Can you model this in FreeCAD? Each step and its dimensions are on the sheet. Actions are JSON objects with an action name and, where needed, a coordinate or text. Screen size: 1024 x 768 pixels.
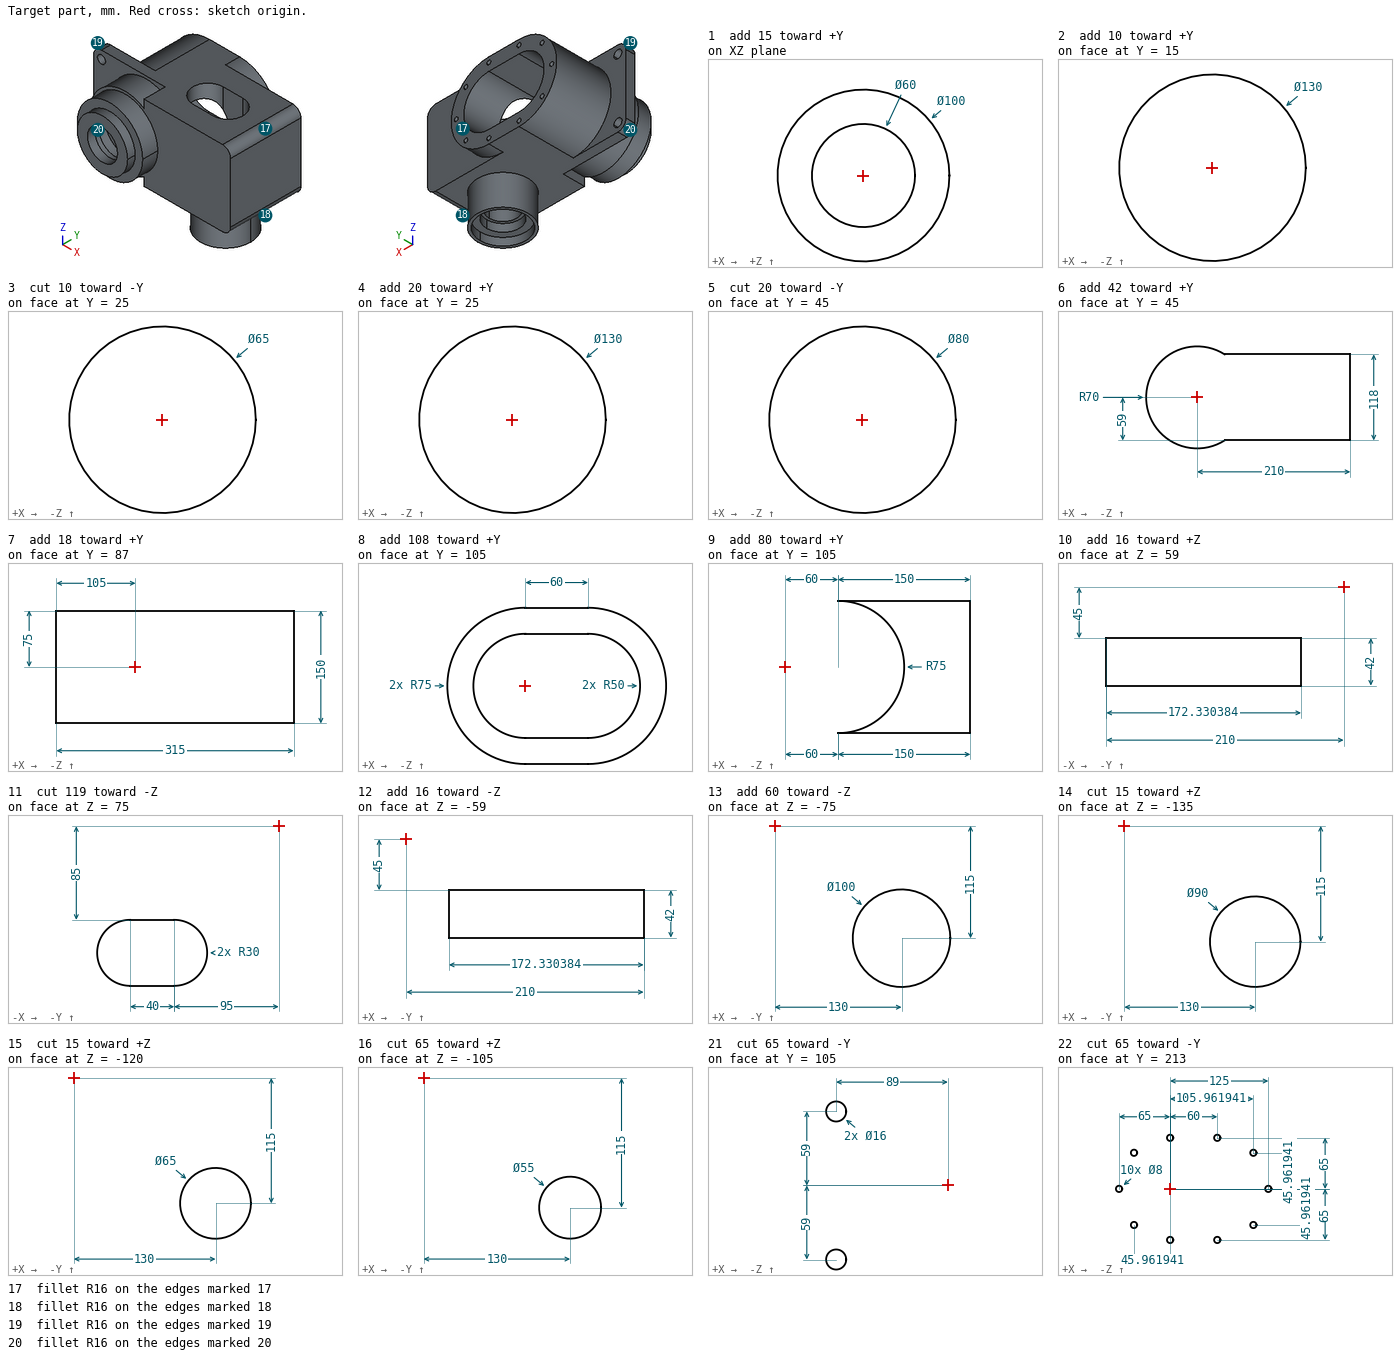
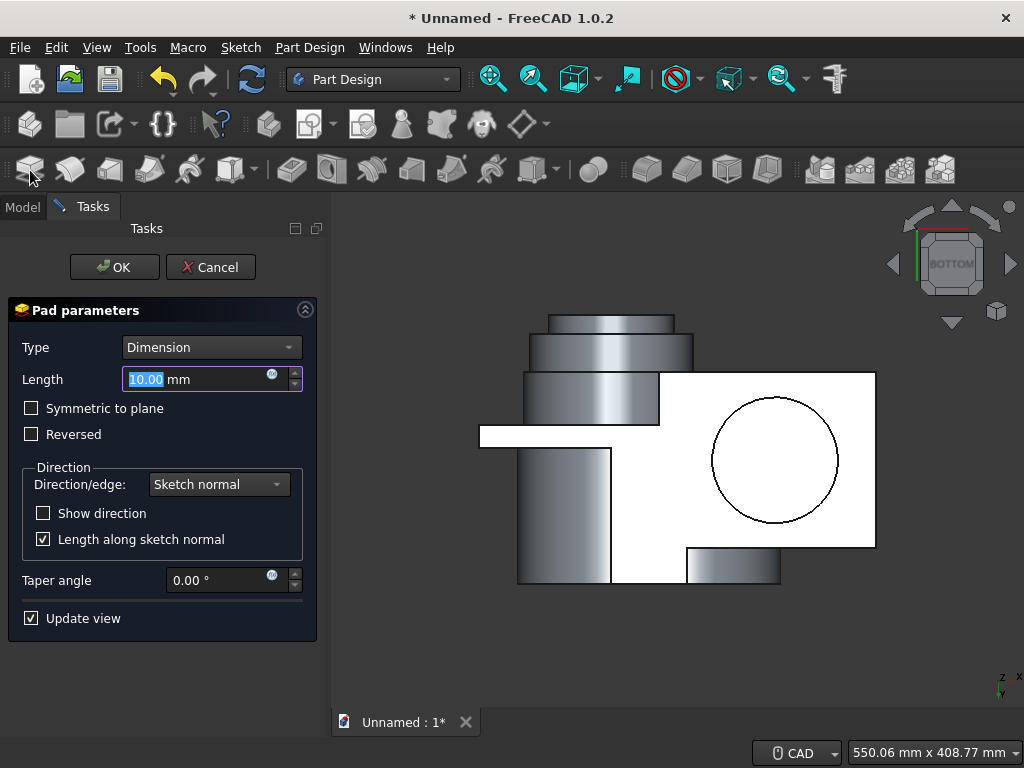
{"action": "type", "text": "60"}
{"action": "key", "text": "Tab"}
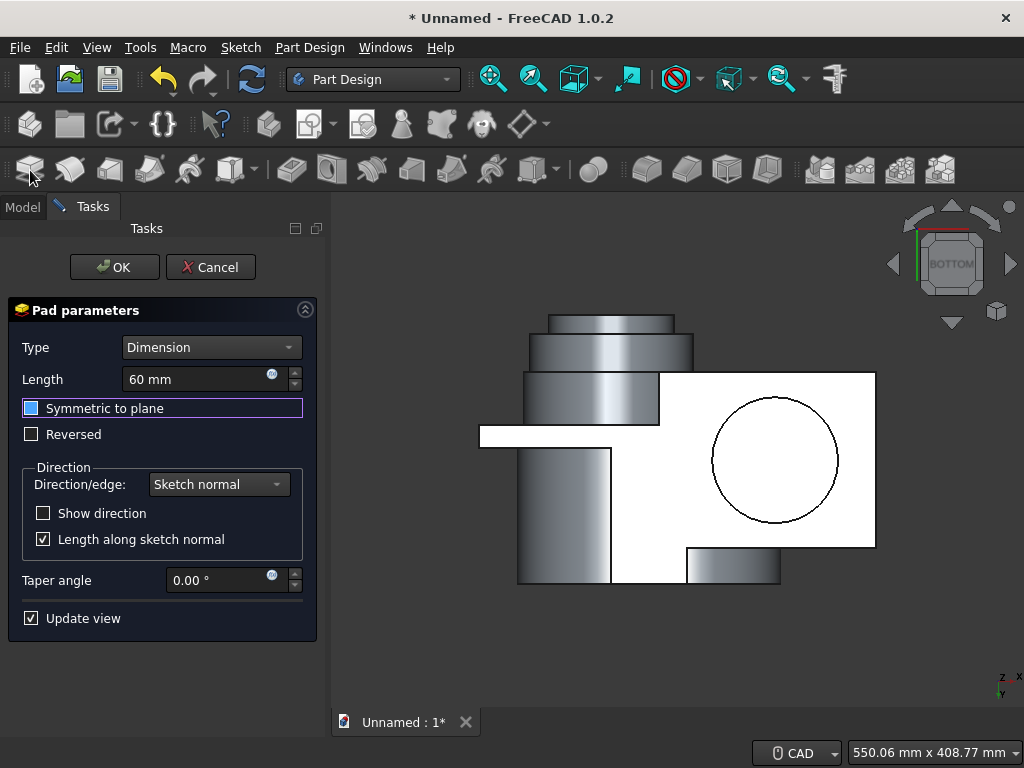
{"action": "left_click", "coordinate": [115, 267]}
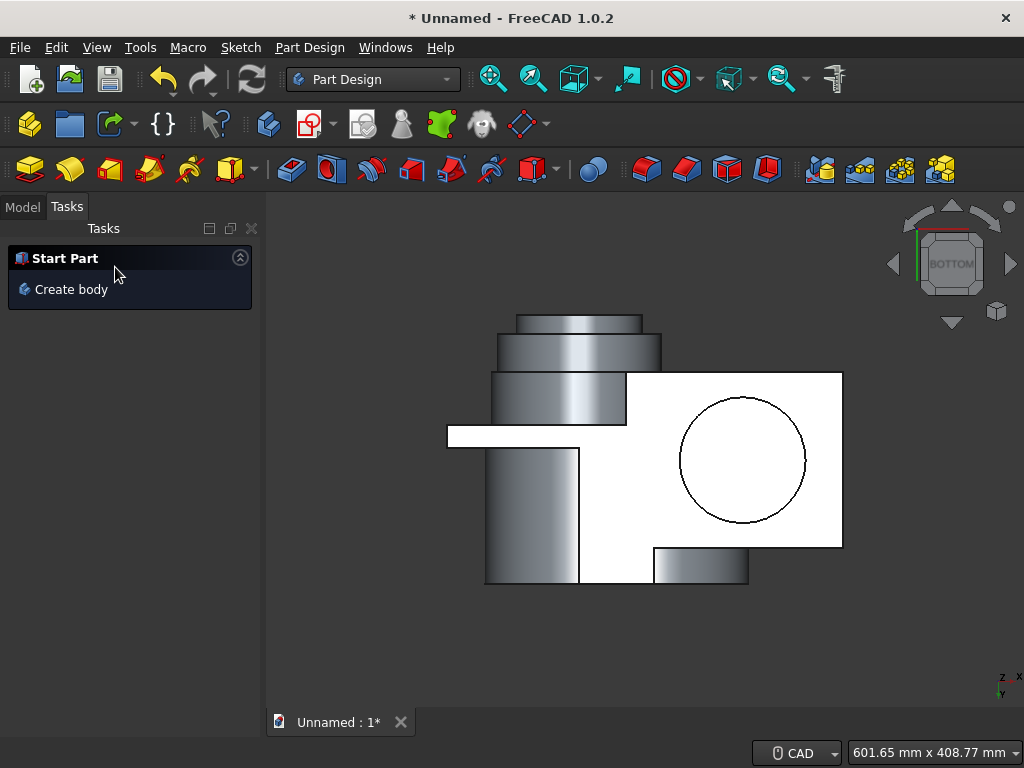
{"action": "left_click", "coordinate": [743, 459]}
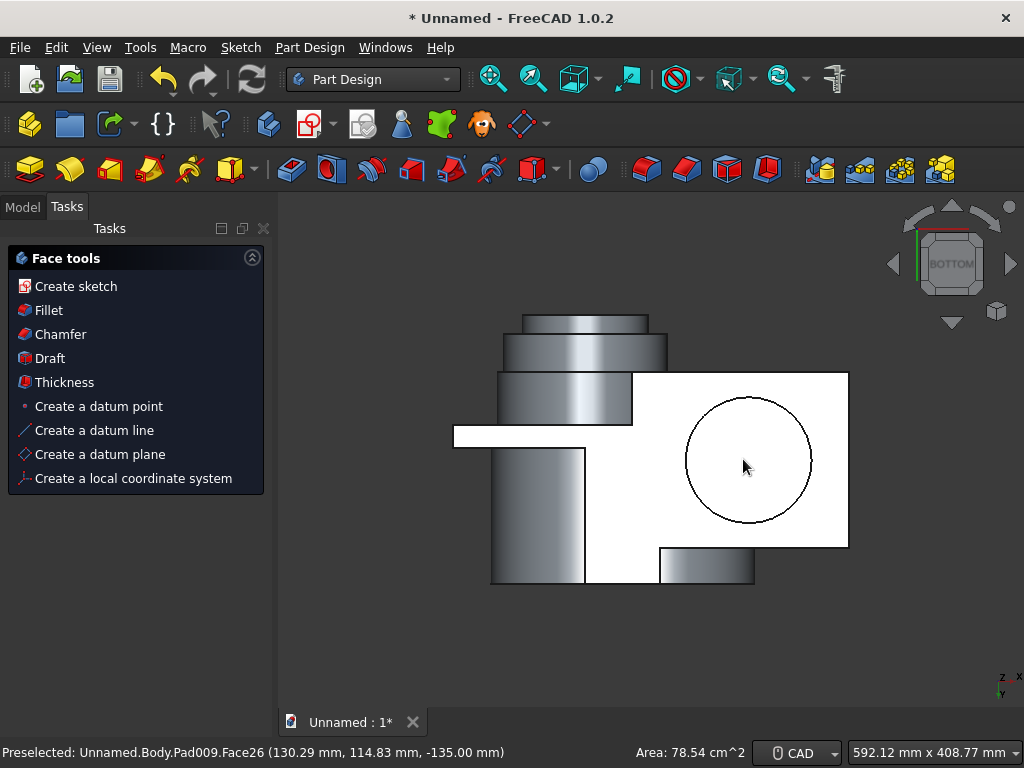
{"action": "left_click", "coordinate": [310, 124]}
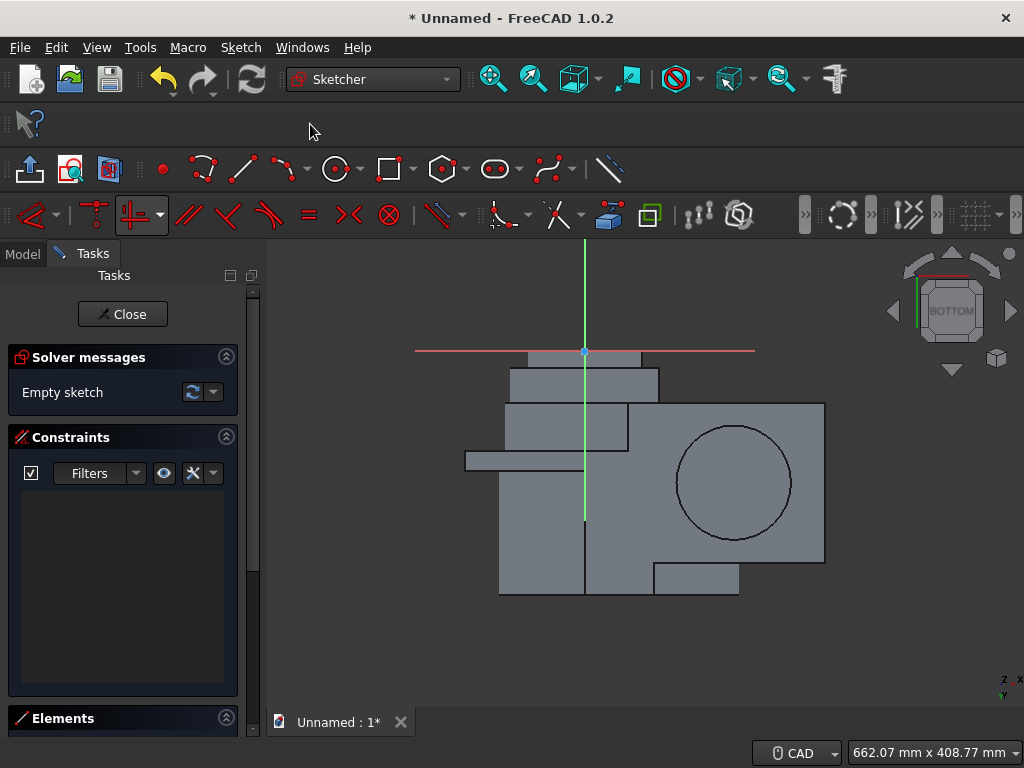
{"action": "scroll", "coordinate": [859, 381], "scroll_direction": "up", "scroll_amount": 2}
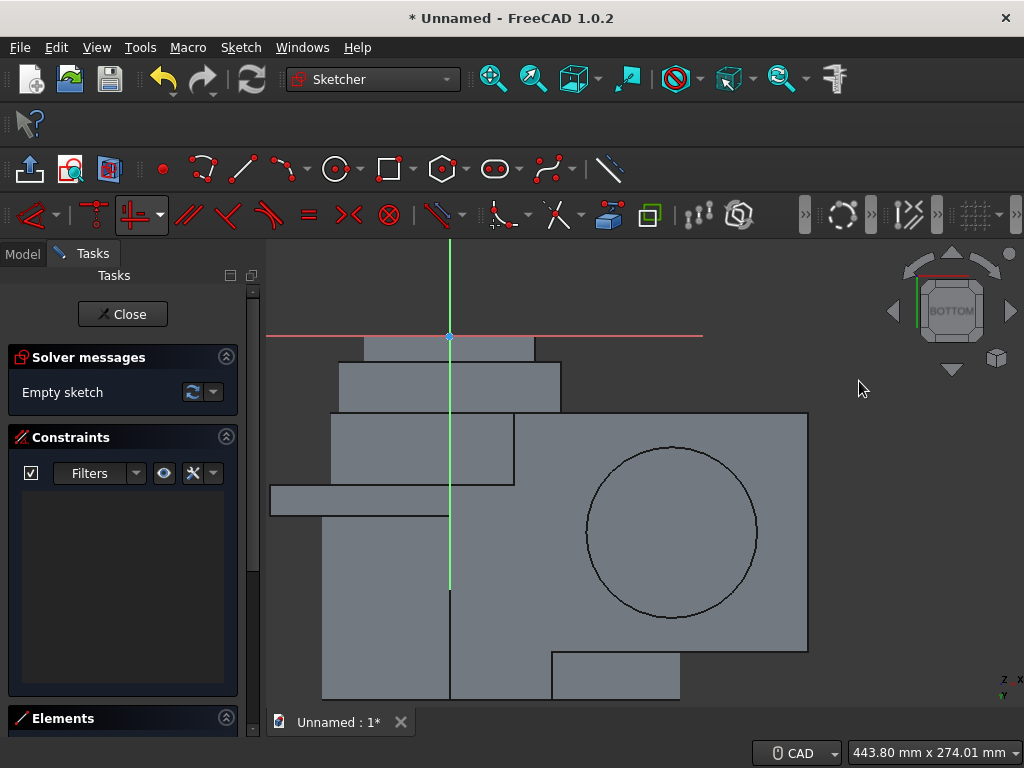
{"action": "left_click", "coordinate": [336, 170]}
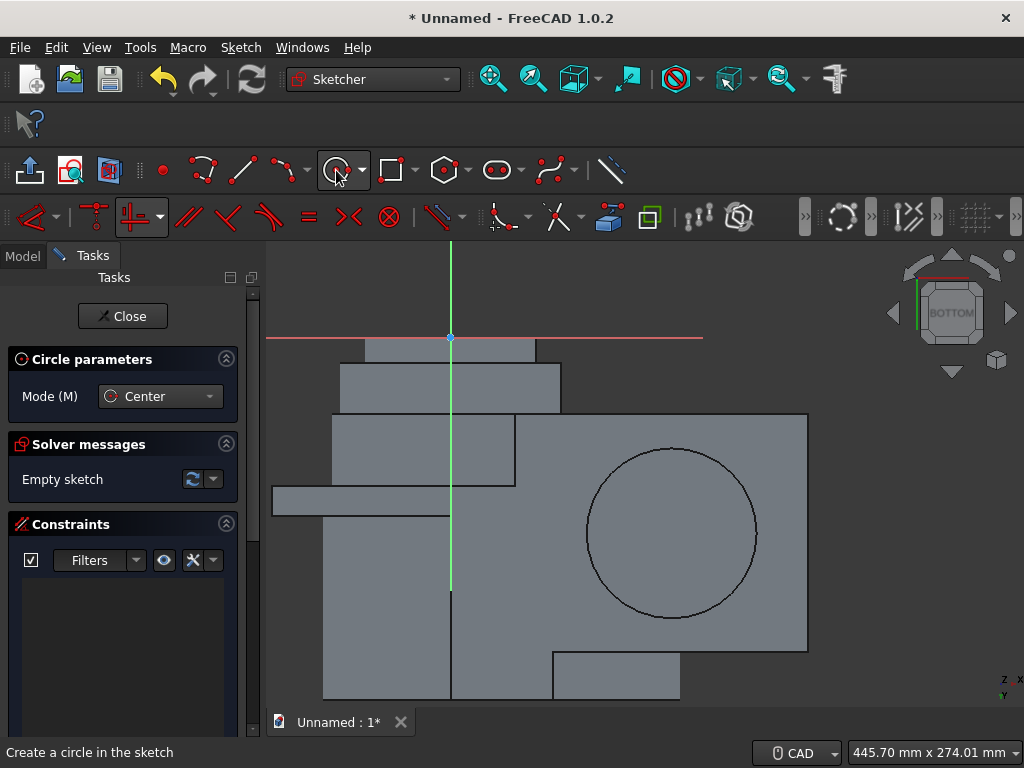
{"action": "left_click", "coordinate": [672, 533]}
{"action": "mouse_move", "coordinate": [726, 479]}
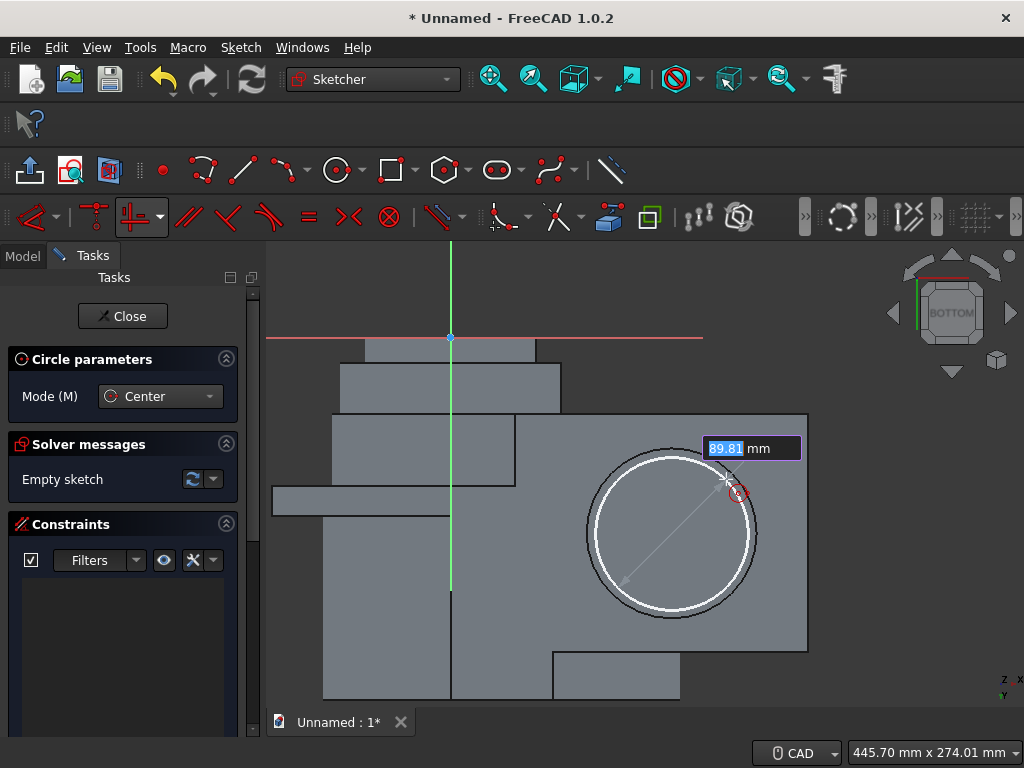
{"action": "type", "text": "90"}
{"action": "key", "text": "Return"}
{"action": "key", "text": "Escape"}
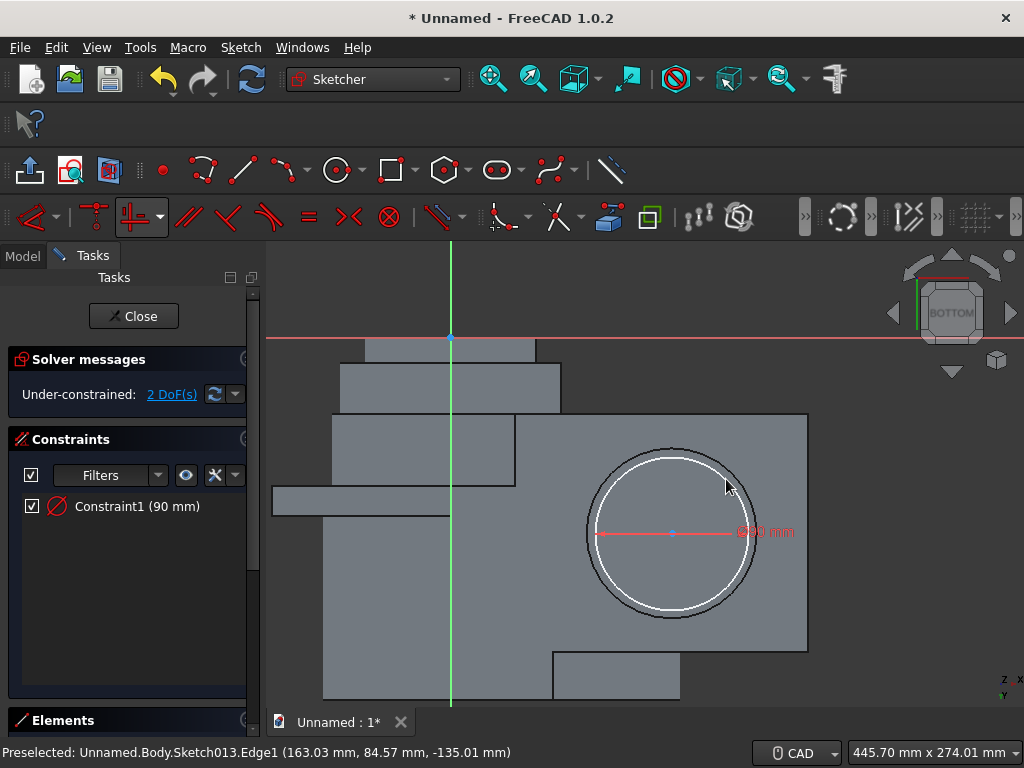
{"action": "left_click", "coordinate": [32, 218]}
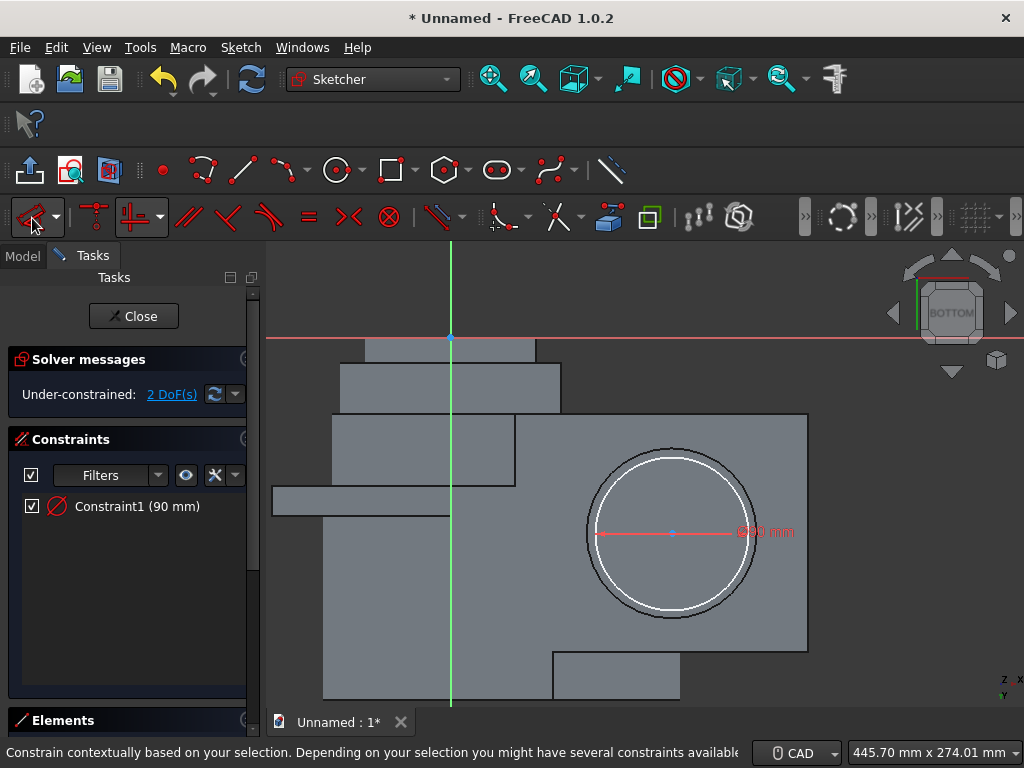
{"action": "left_click", "coordinate": [672, 534]}
{"action": "left_click", "coordinate": [561, 304]}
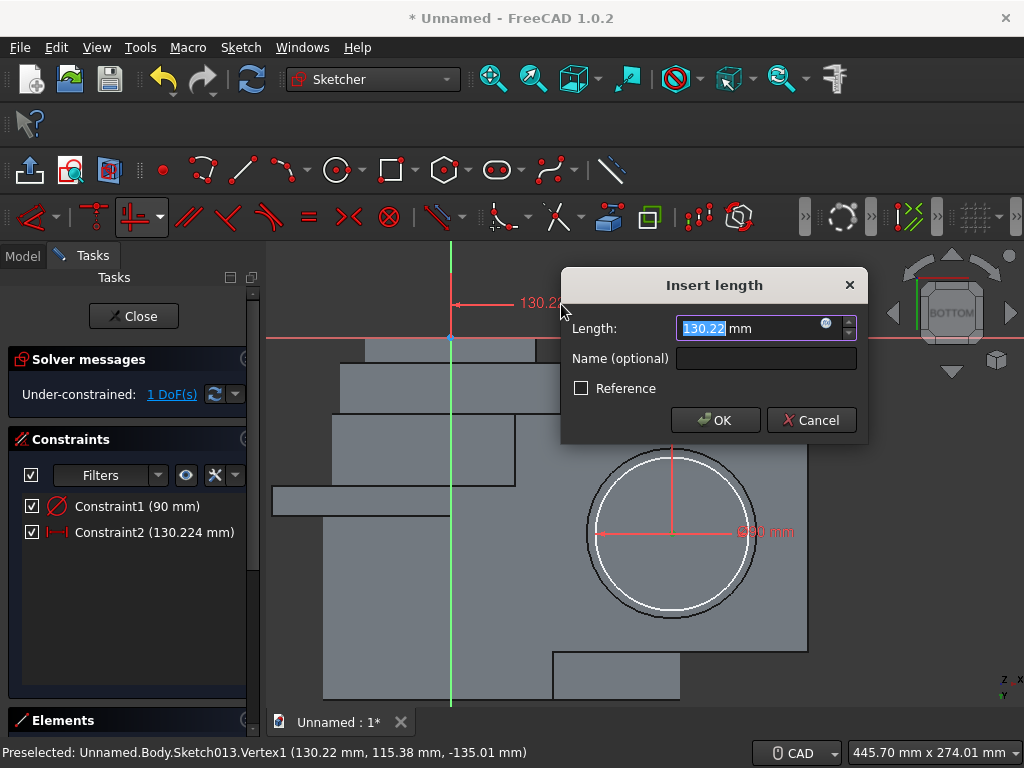
{"action": "type", "text": "130"}
{"action": "key", "text": "Return"}